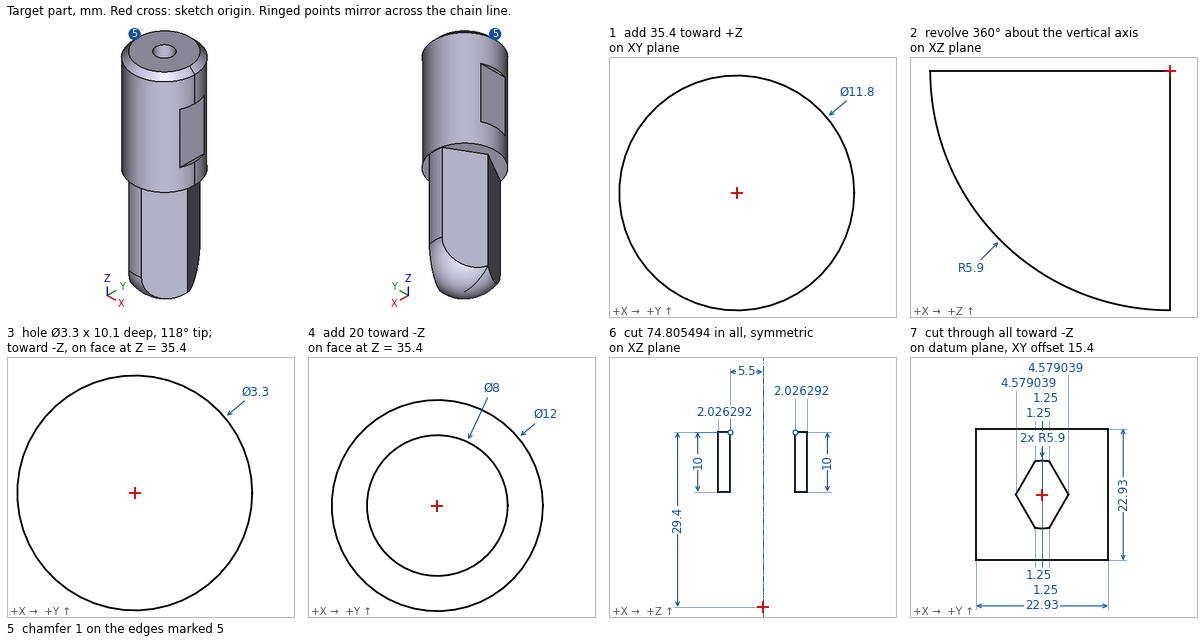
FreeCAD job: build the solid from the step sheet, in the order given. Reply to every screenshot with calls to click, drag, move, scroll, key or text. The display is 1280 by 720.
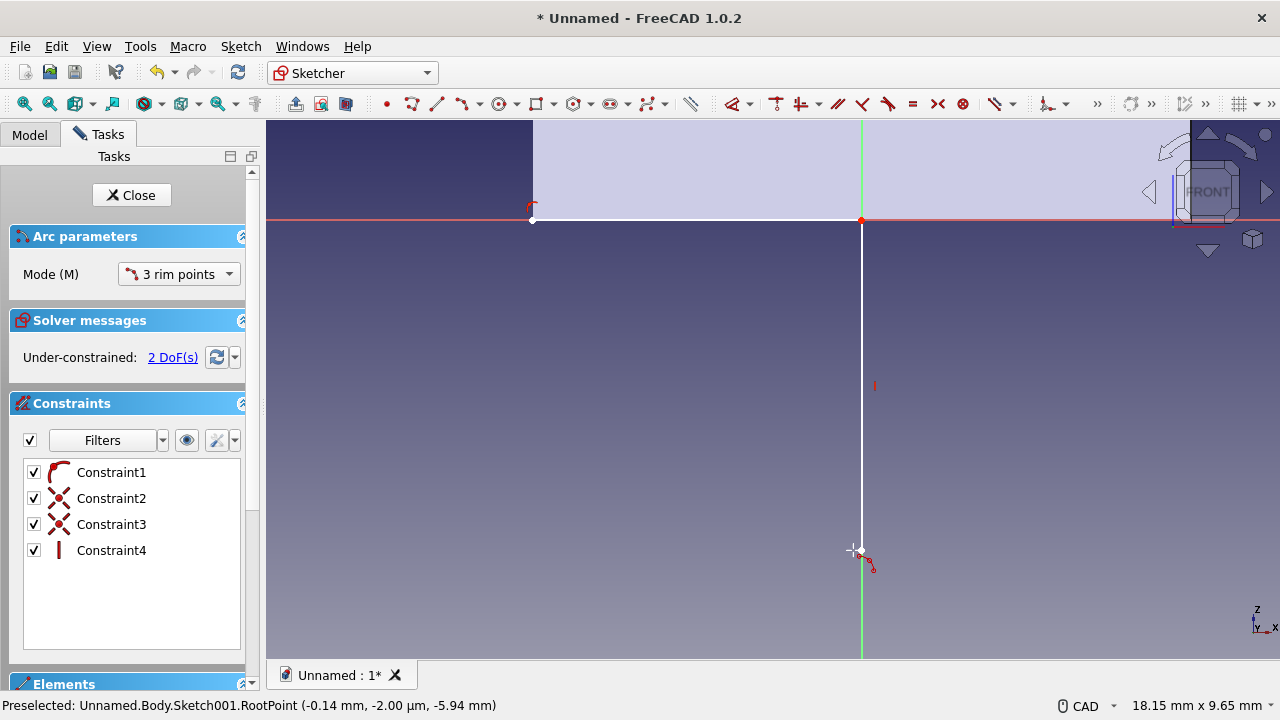
click(862, 551)
click(532, 220)
click(629, 453)
key(Escape)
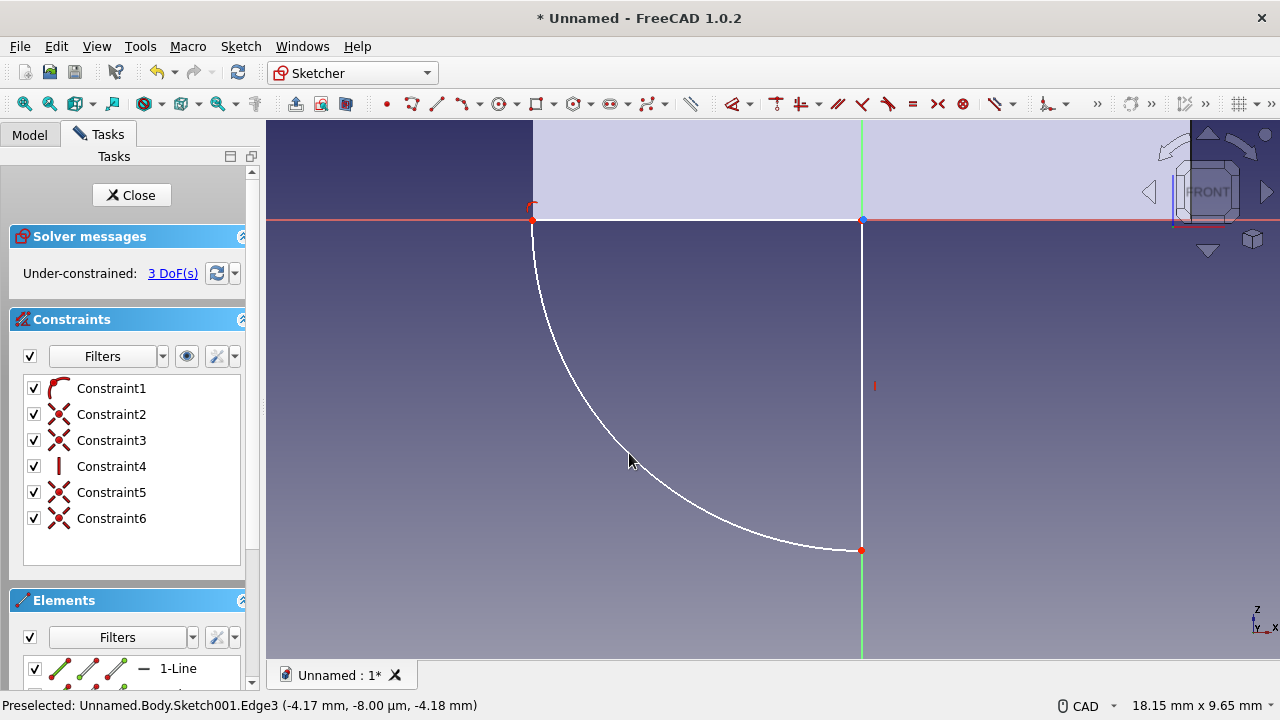
scroll(862, 220, up, 20)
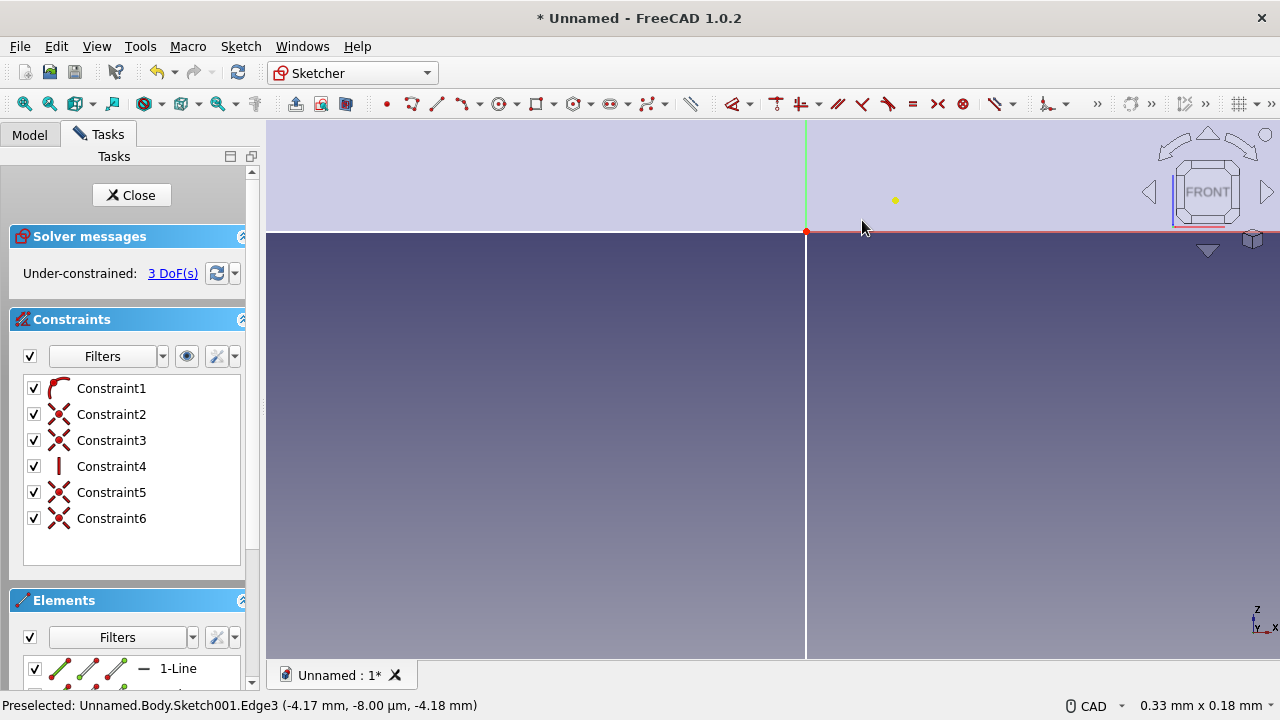
drag(796, 190, 905, 242)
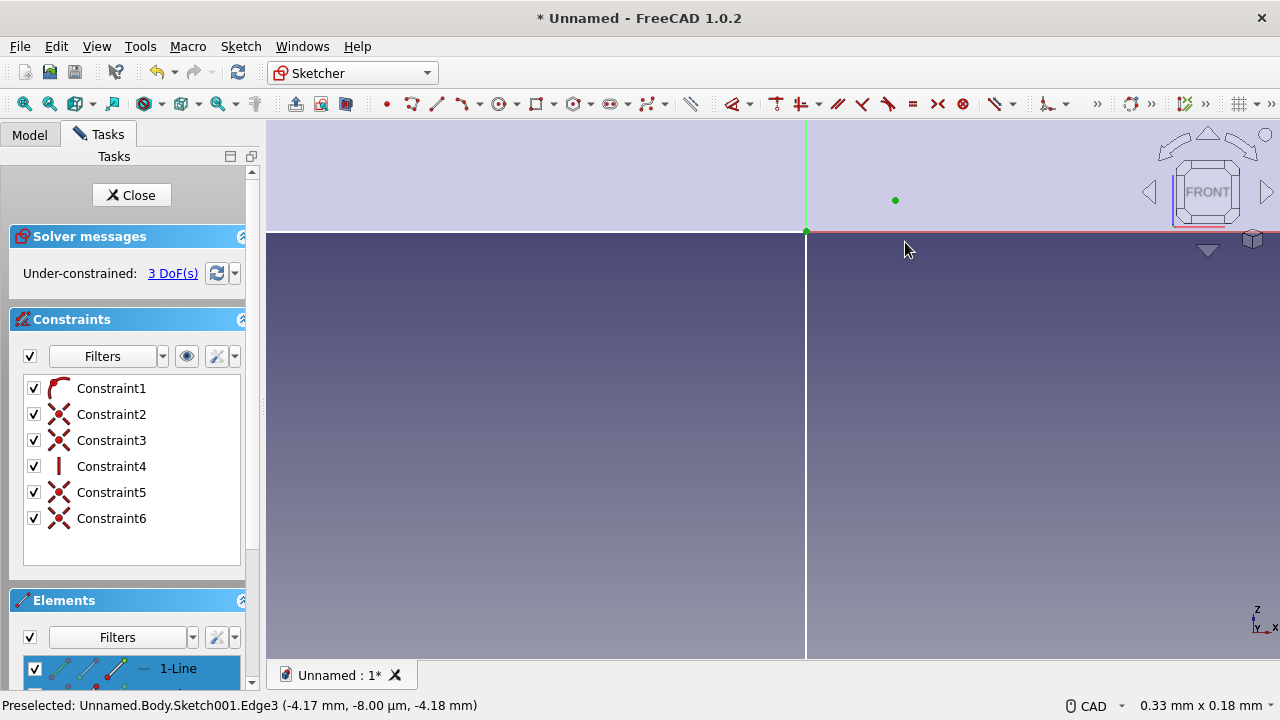
key(c)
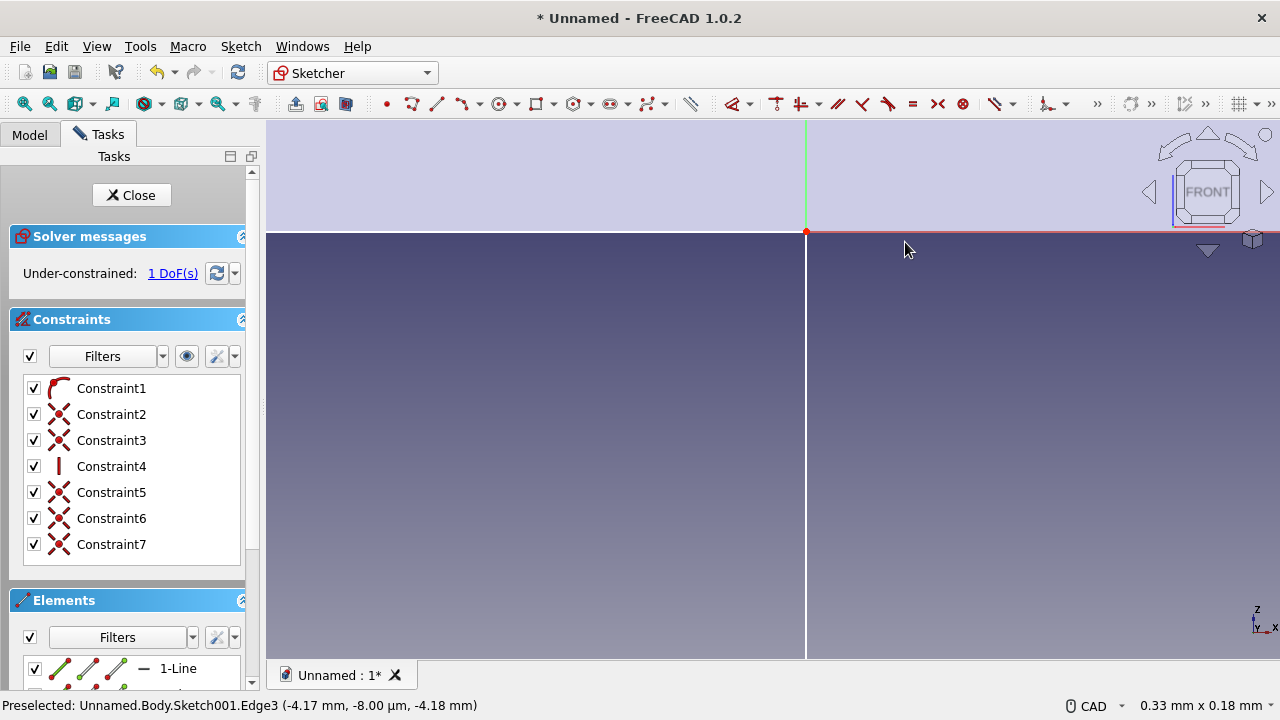
key(d)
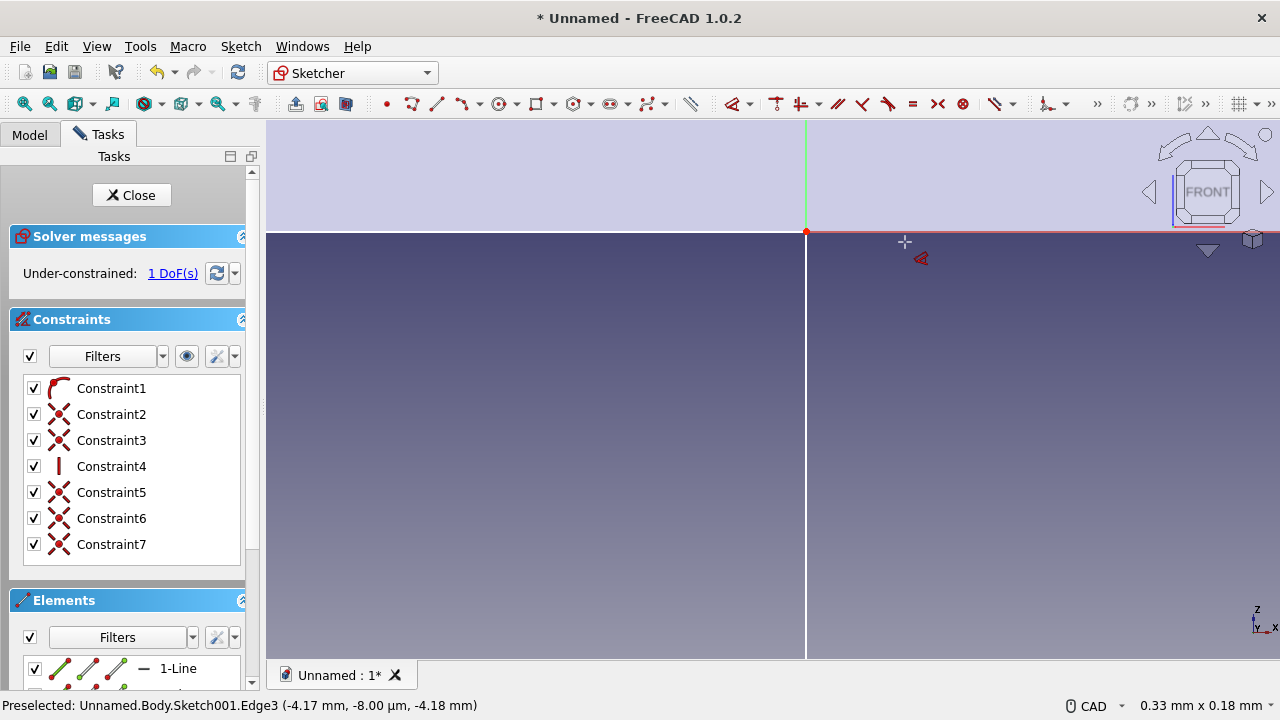
scroll(704, 390, down, 15)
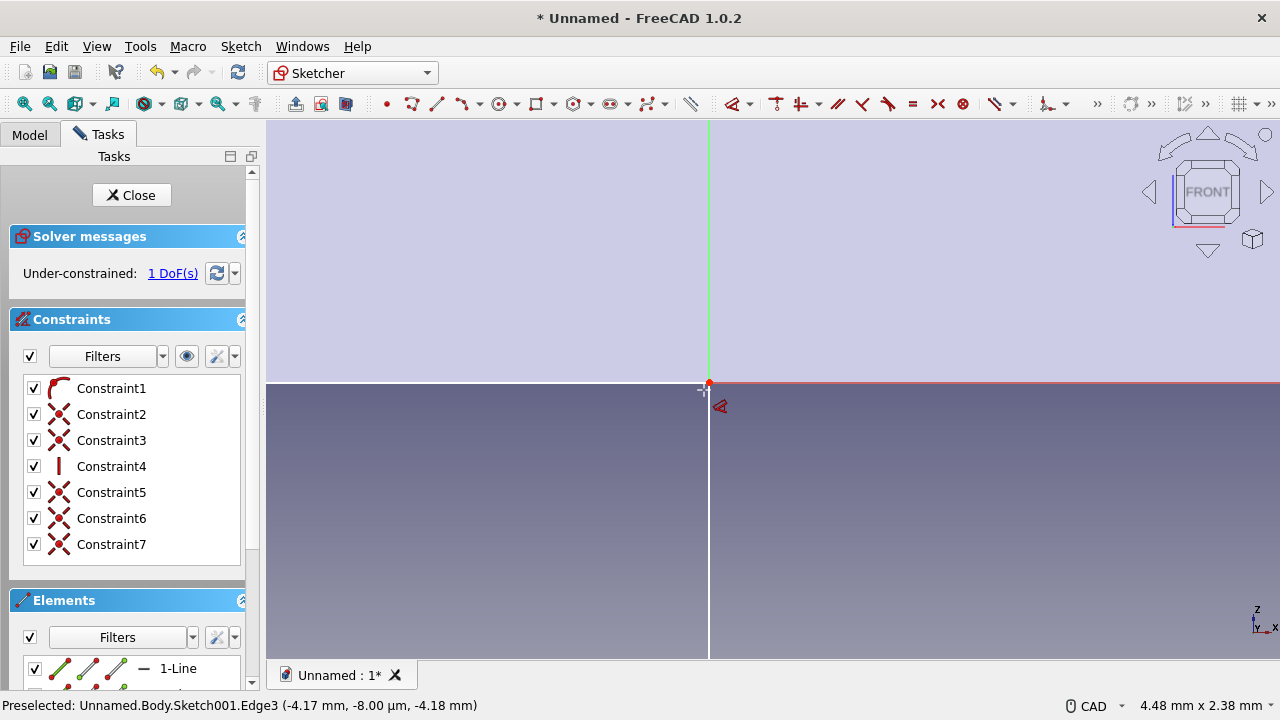
scroll(962, 148, down, 5)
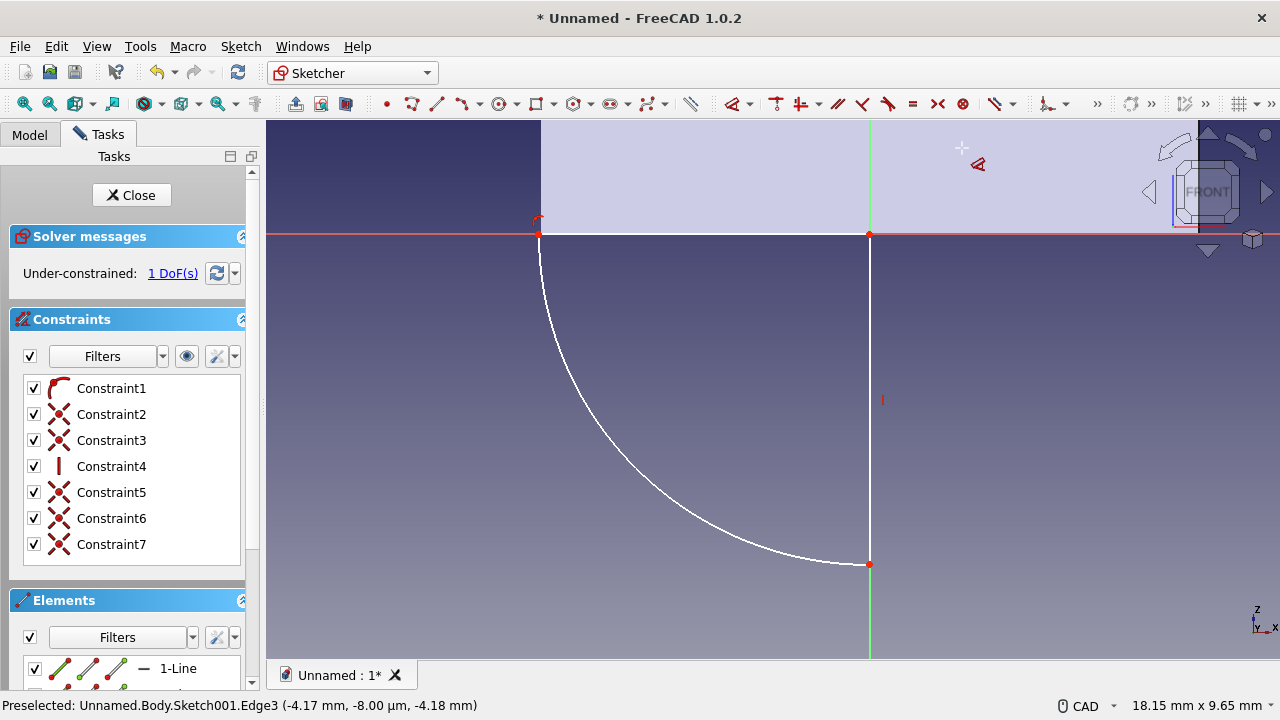
click(575, 384)
click(546, 398)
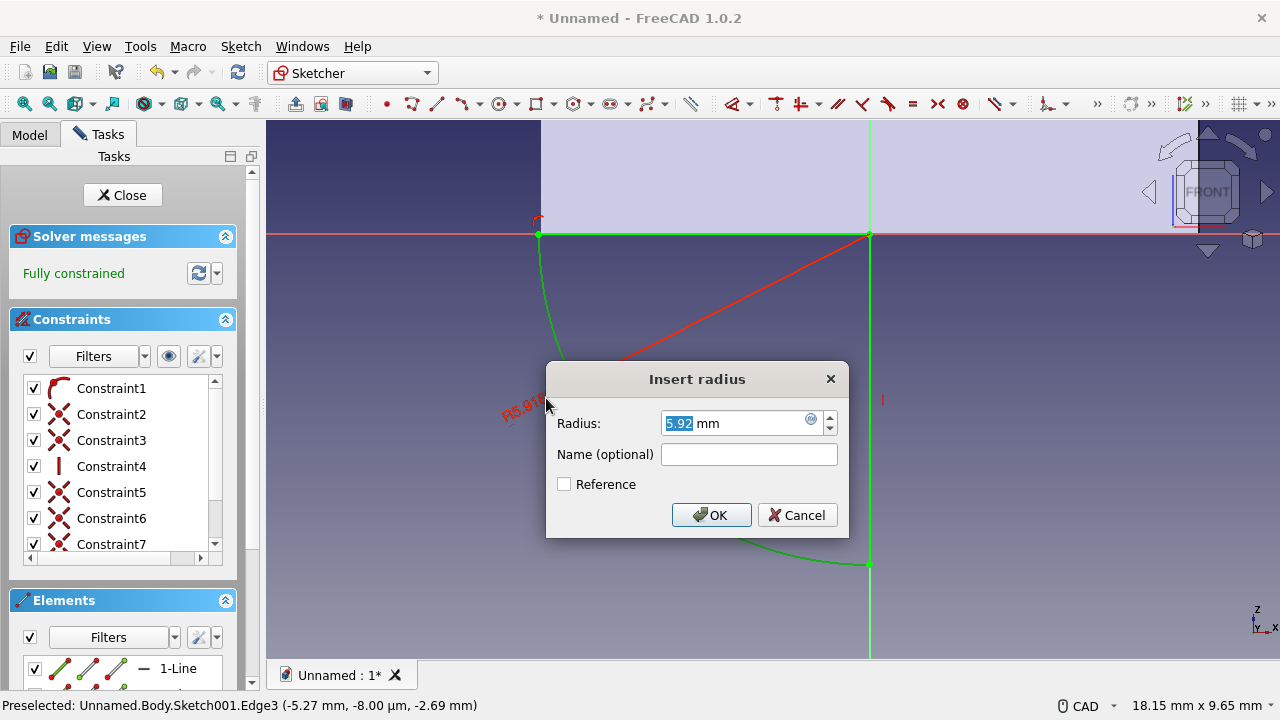
text(5.9)
key(Return)
key(Escape)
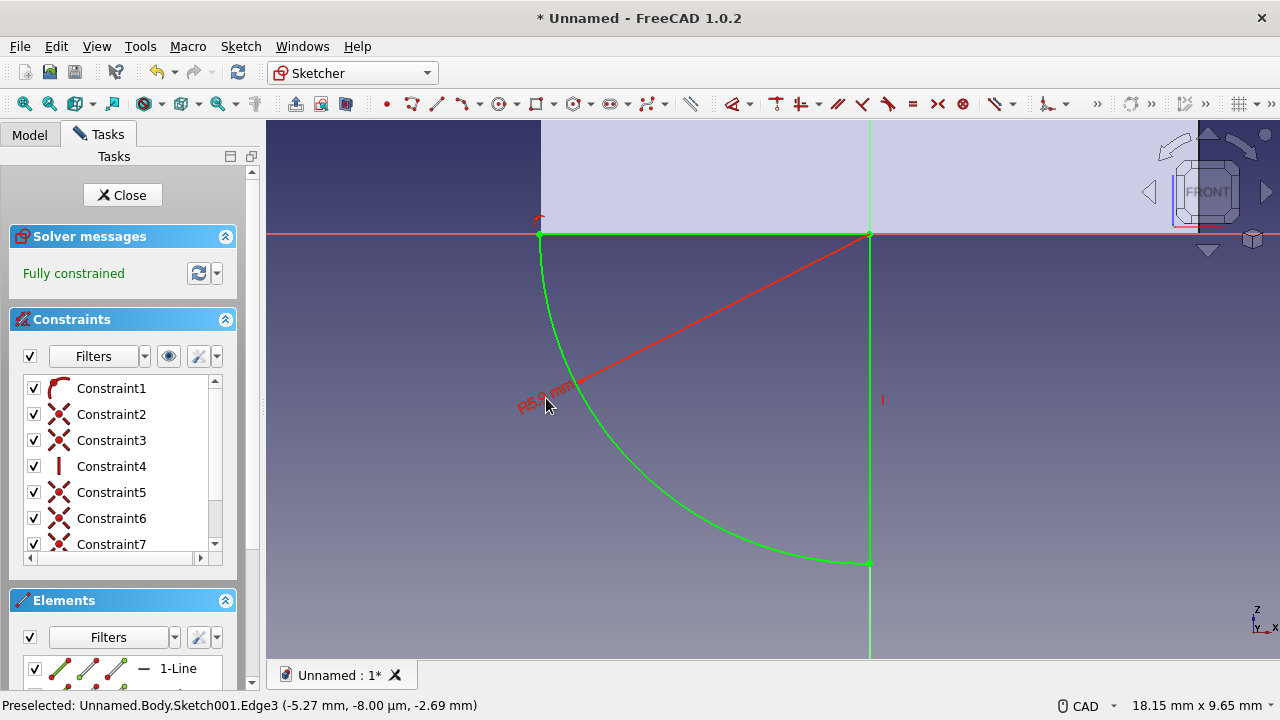
click(123, 195)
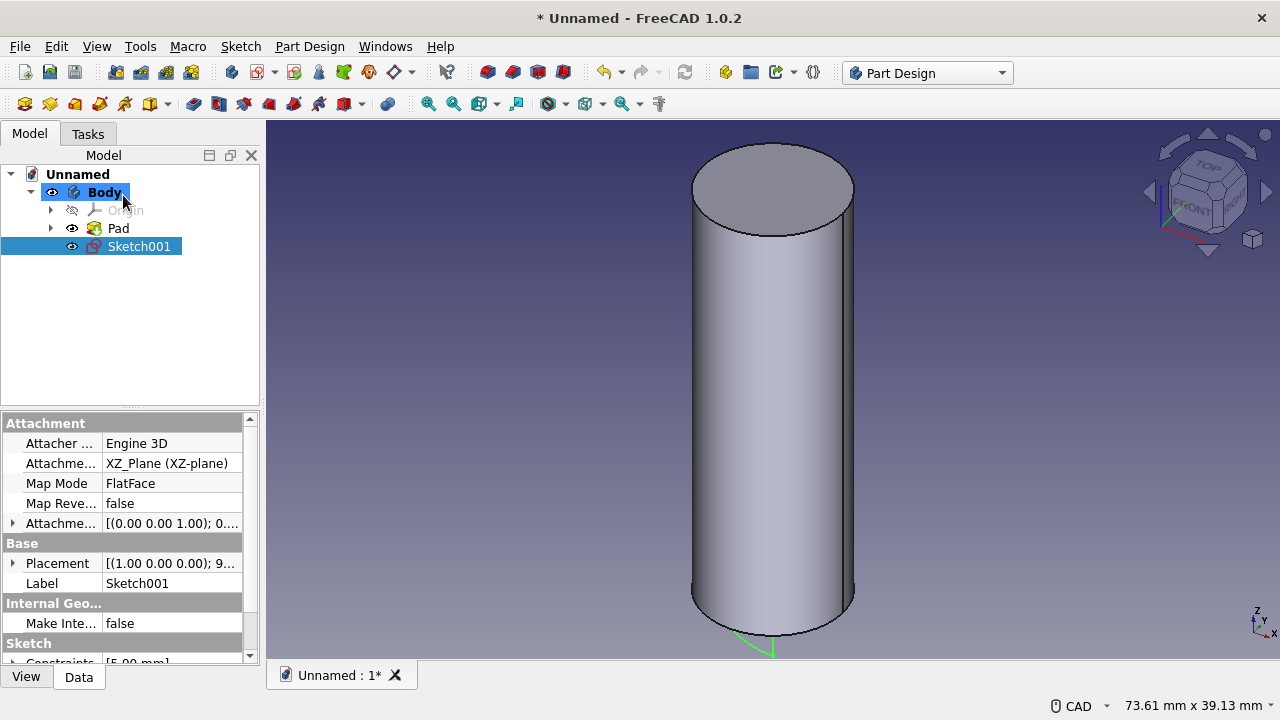
click(50, 104)